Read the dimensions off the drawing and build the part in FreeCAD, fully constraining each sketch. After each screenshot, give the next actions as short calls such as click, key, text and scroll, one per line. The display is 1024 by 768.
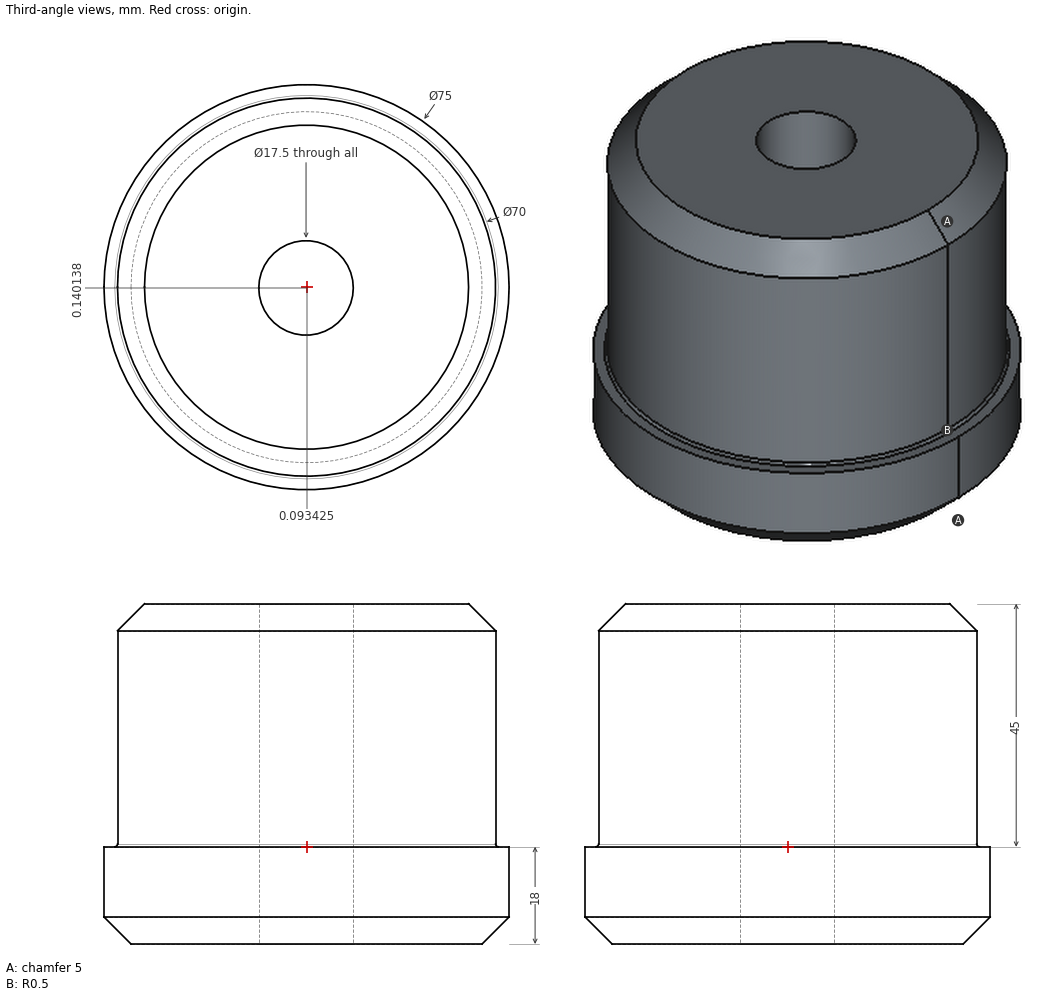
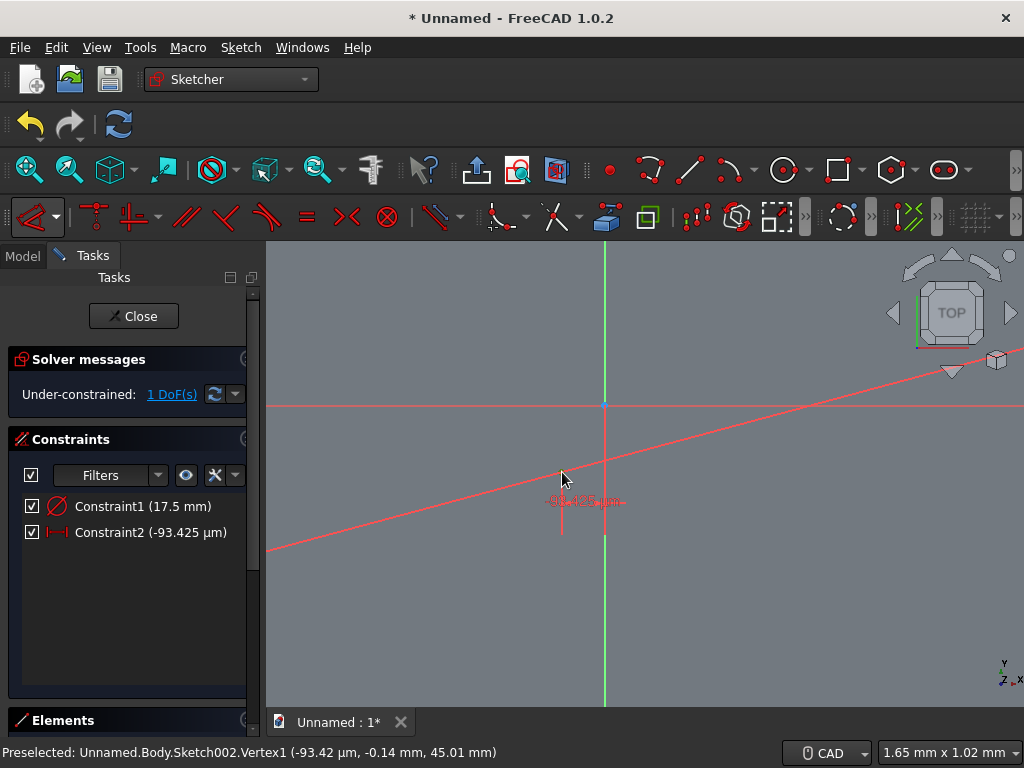
key(i)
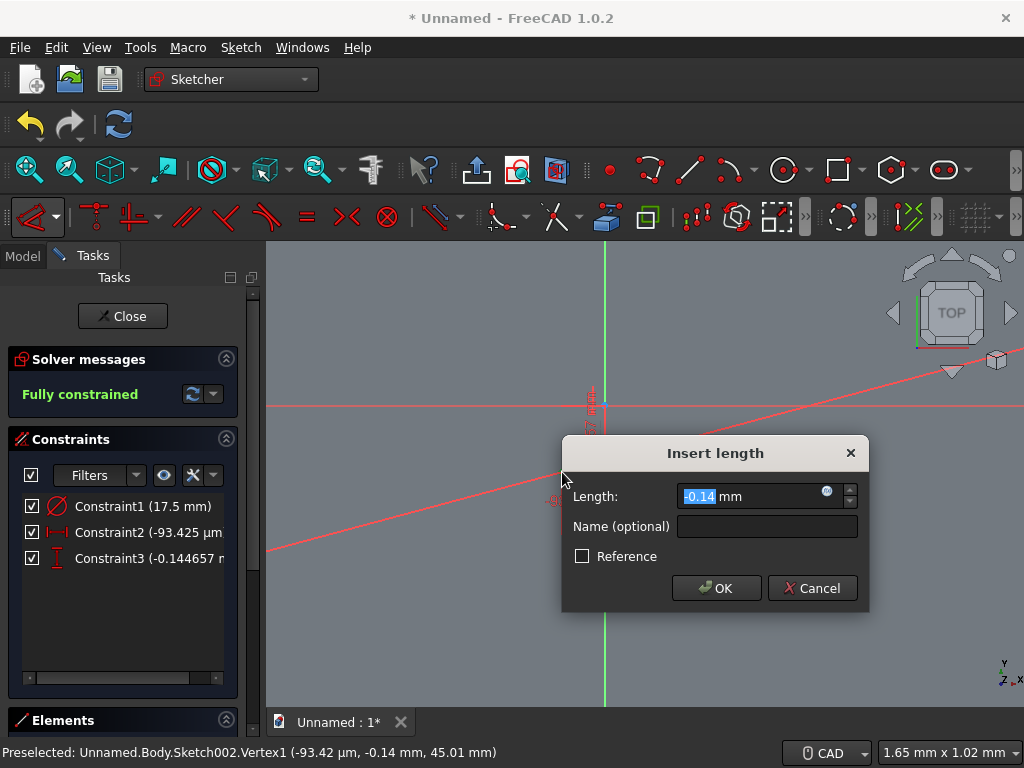
text(-0.140138)
key(Return)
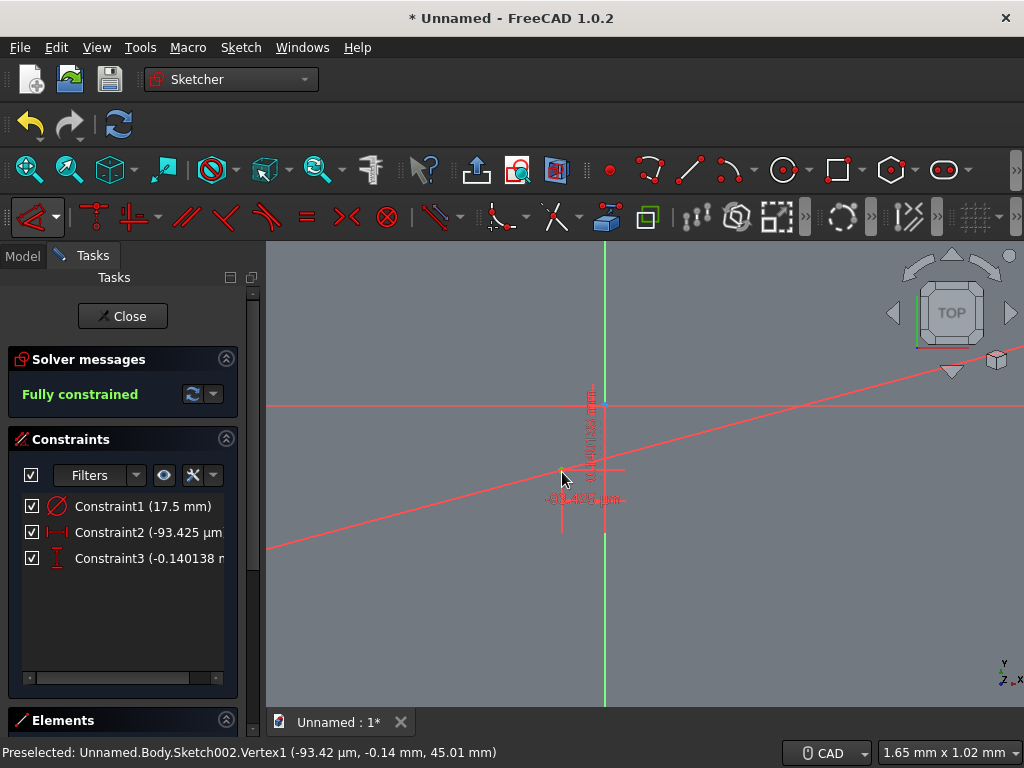
click(123, 316)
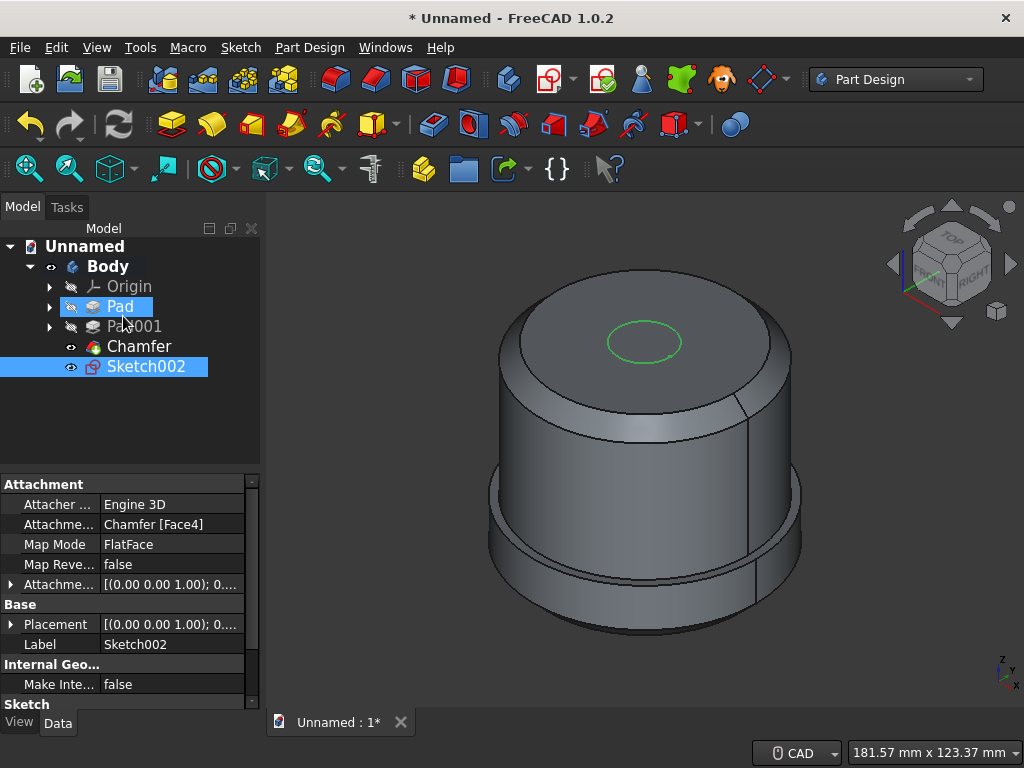
click(474, 124)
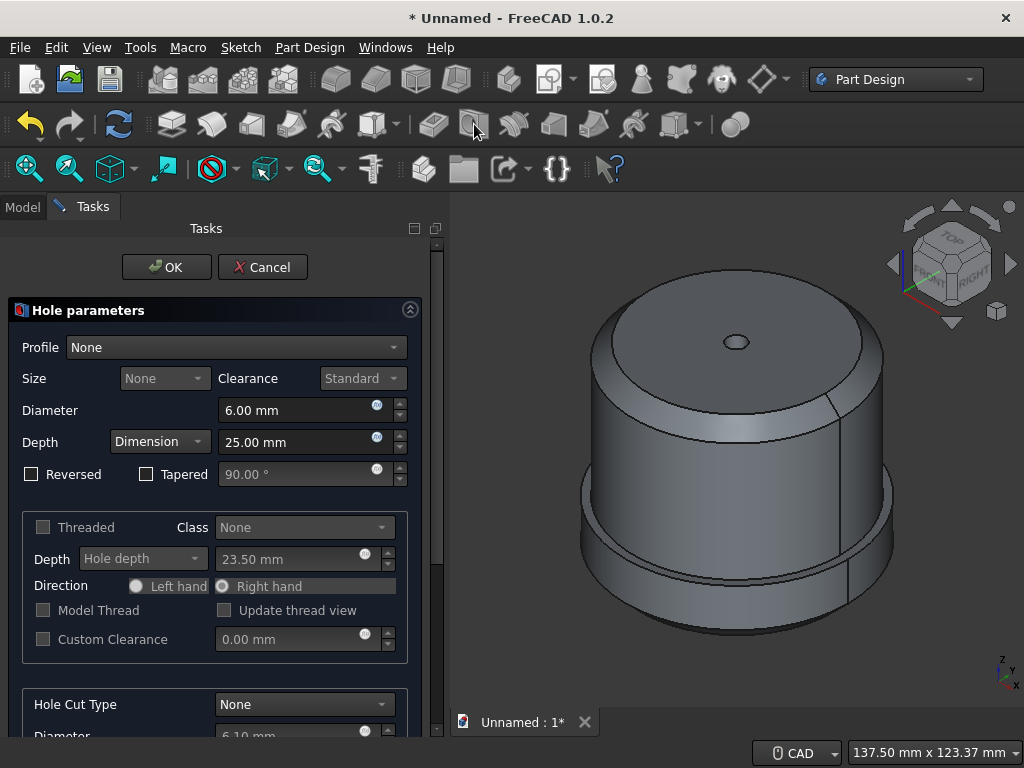
triple_click(305, 410)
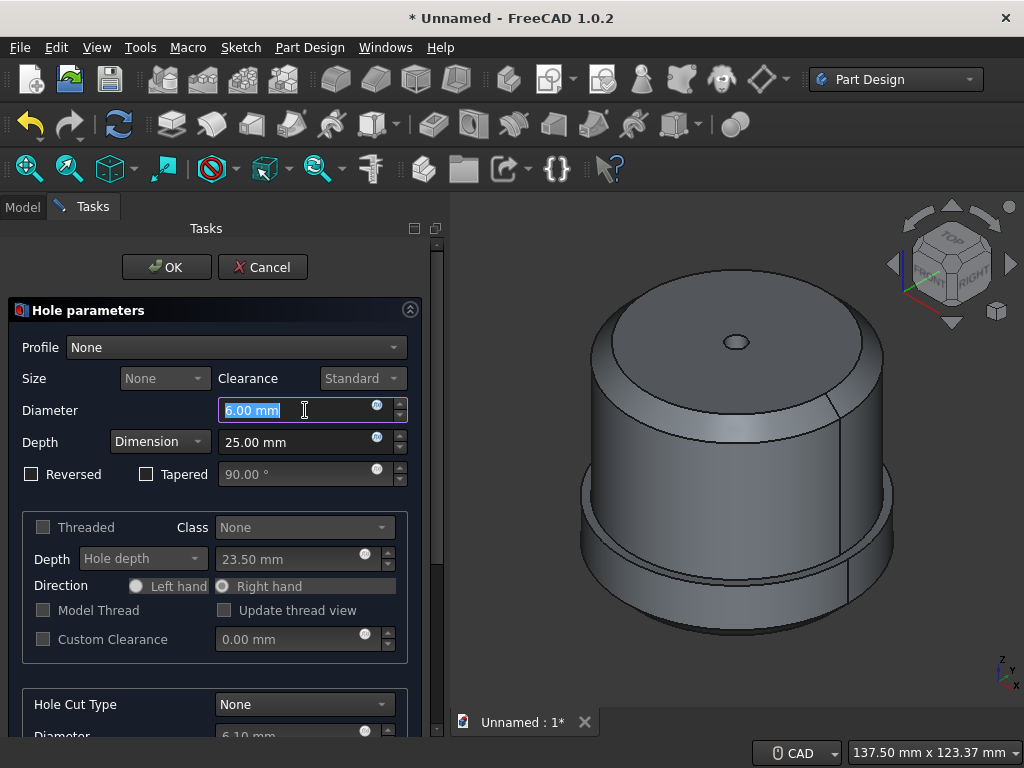
text(17.5)
key(Tab)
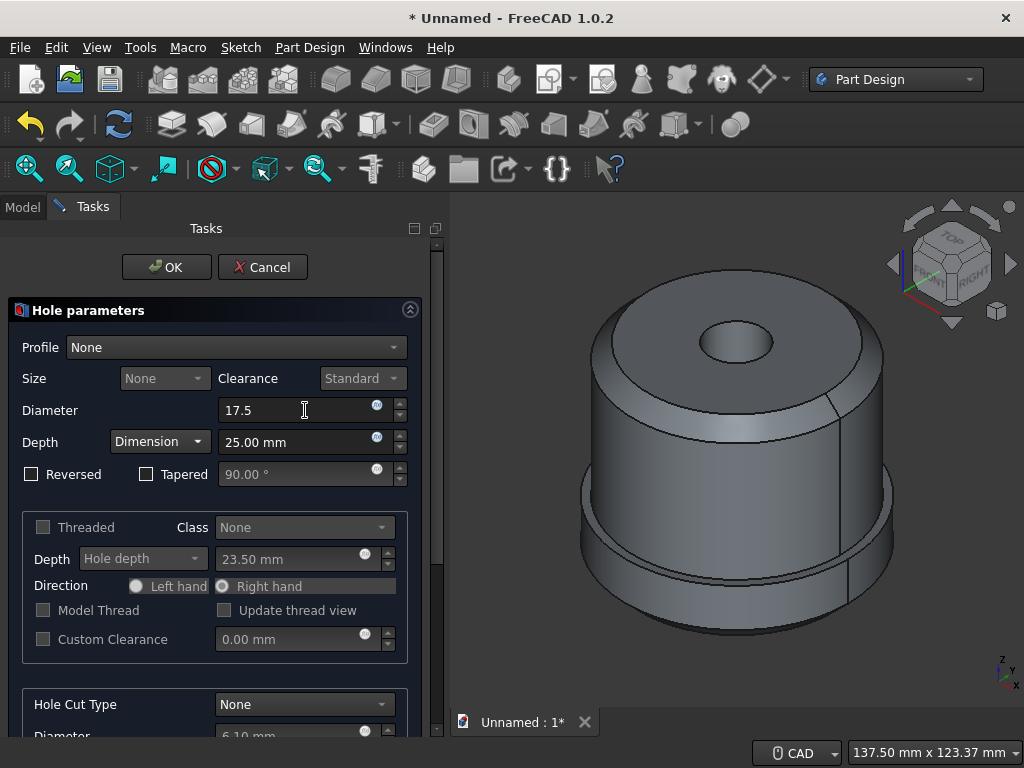
click(161, 442)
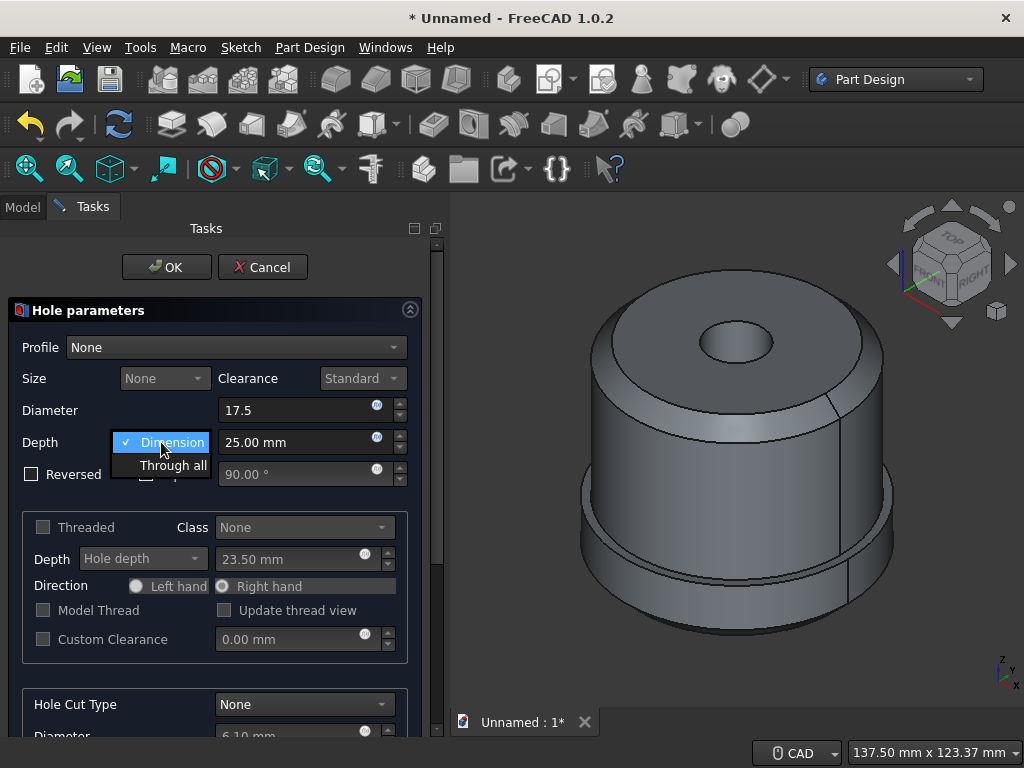
click(160, 466)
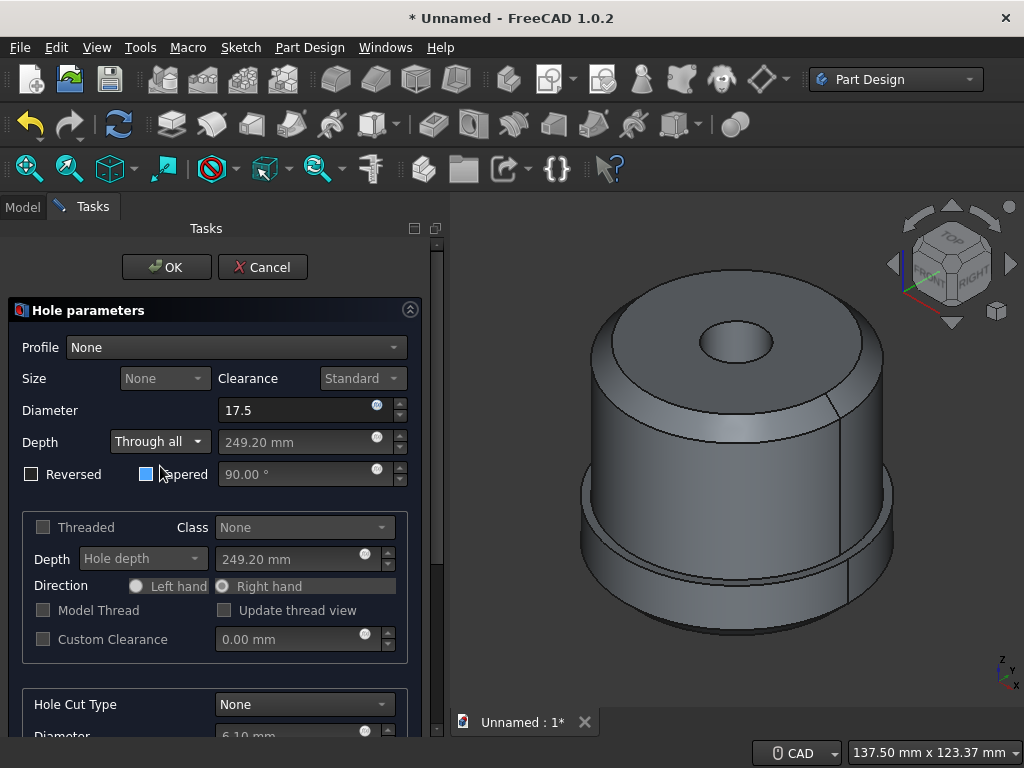
click(167, 267)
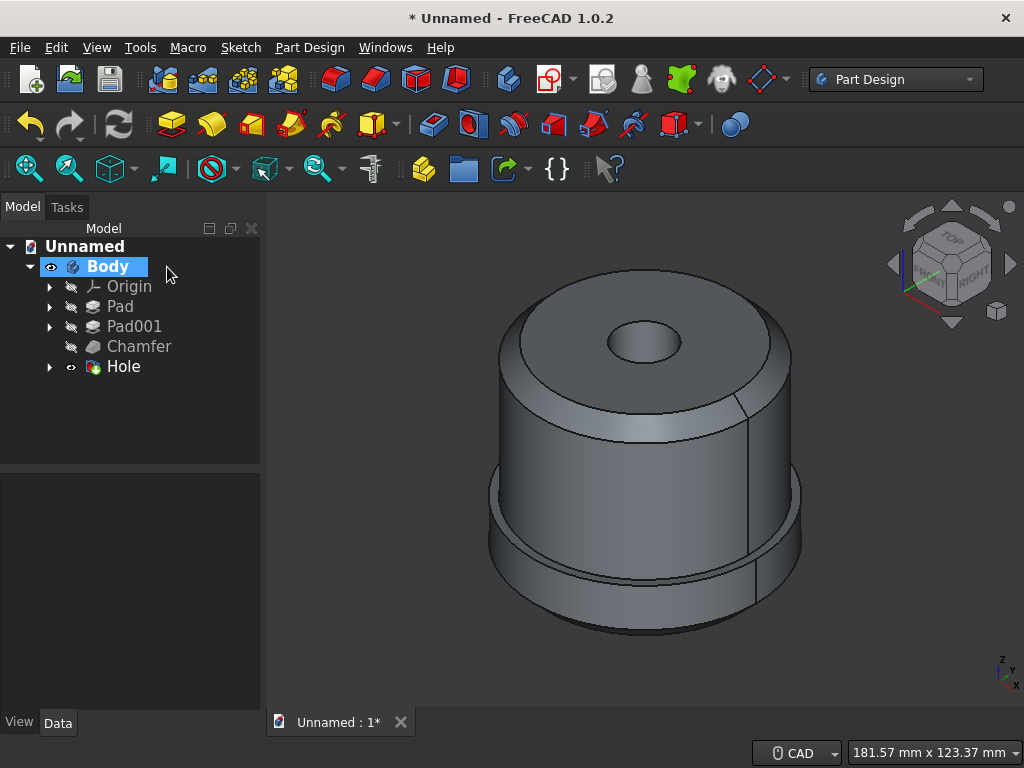
key(2)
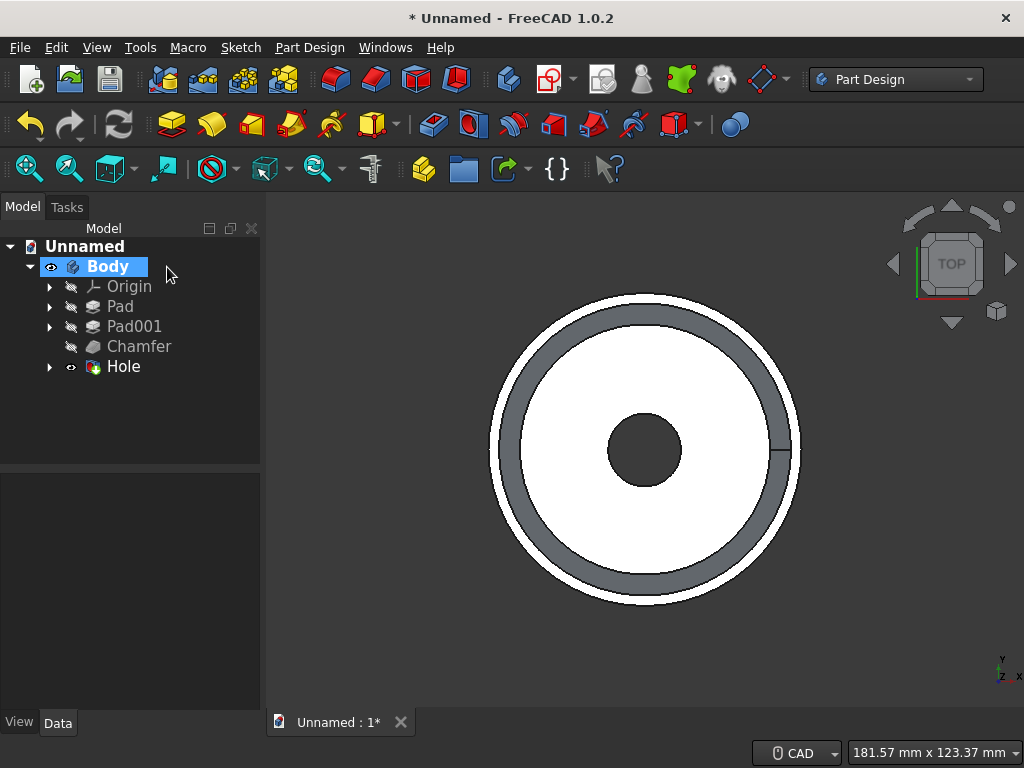
key(0)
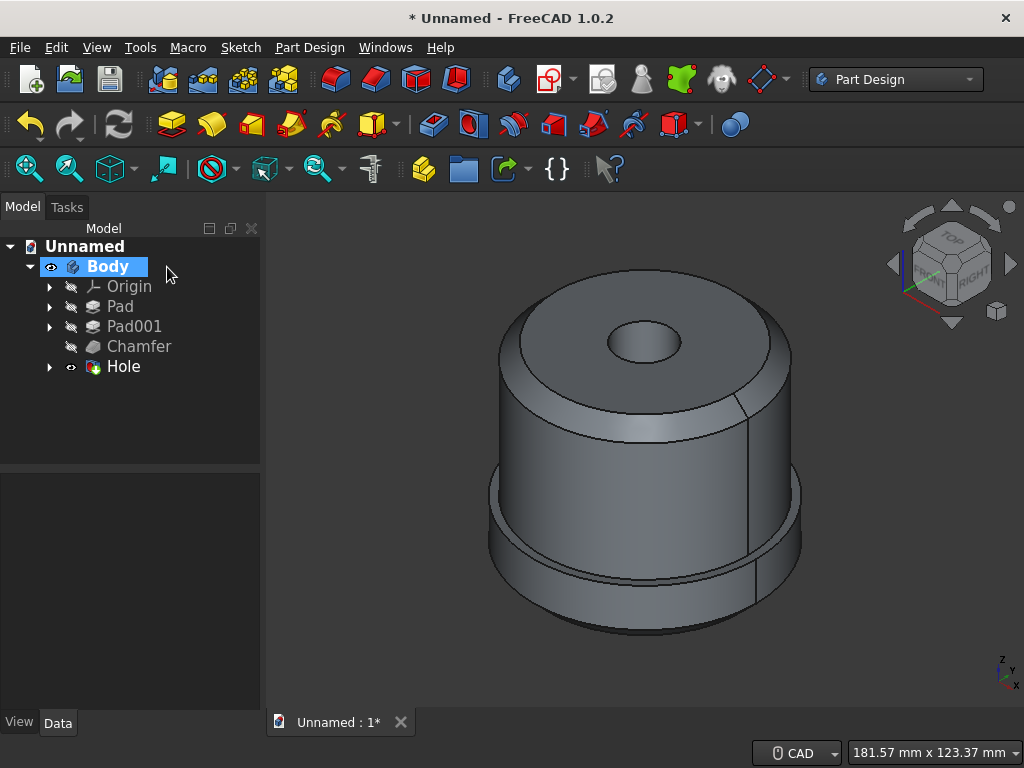
key(1)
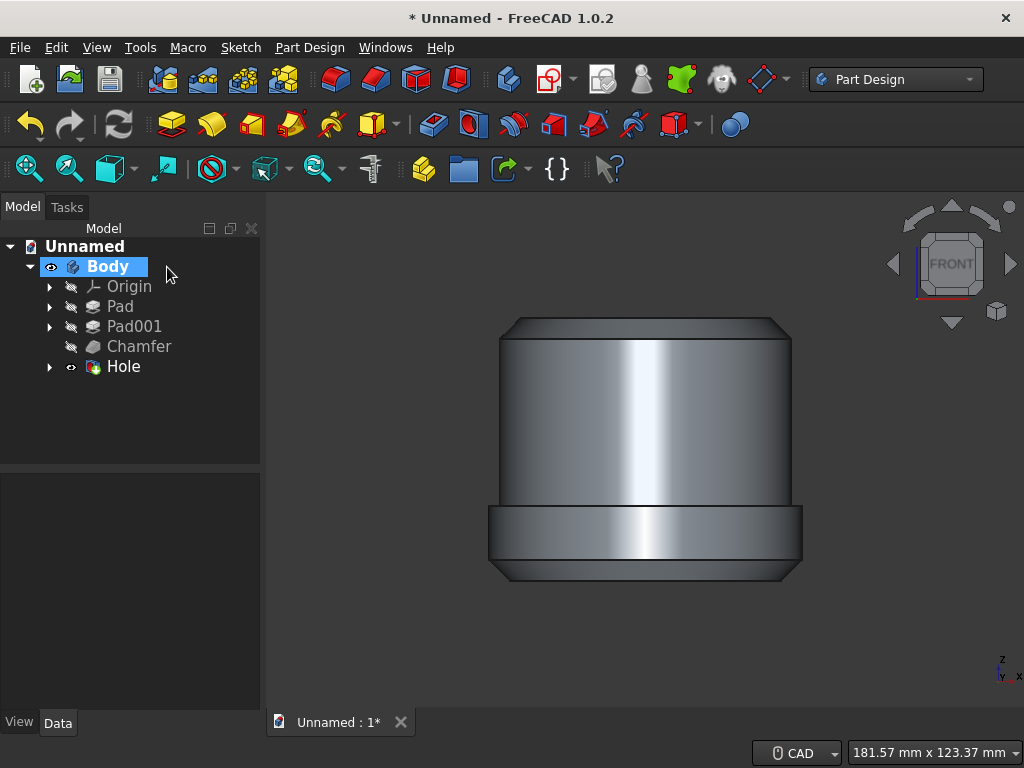
key(3)